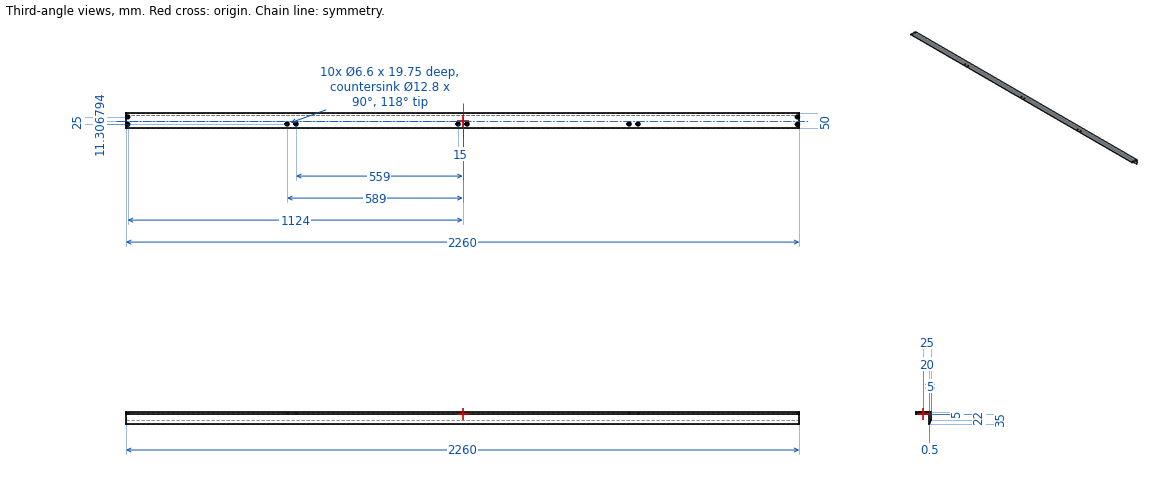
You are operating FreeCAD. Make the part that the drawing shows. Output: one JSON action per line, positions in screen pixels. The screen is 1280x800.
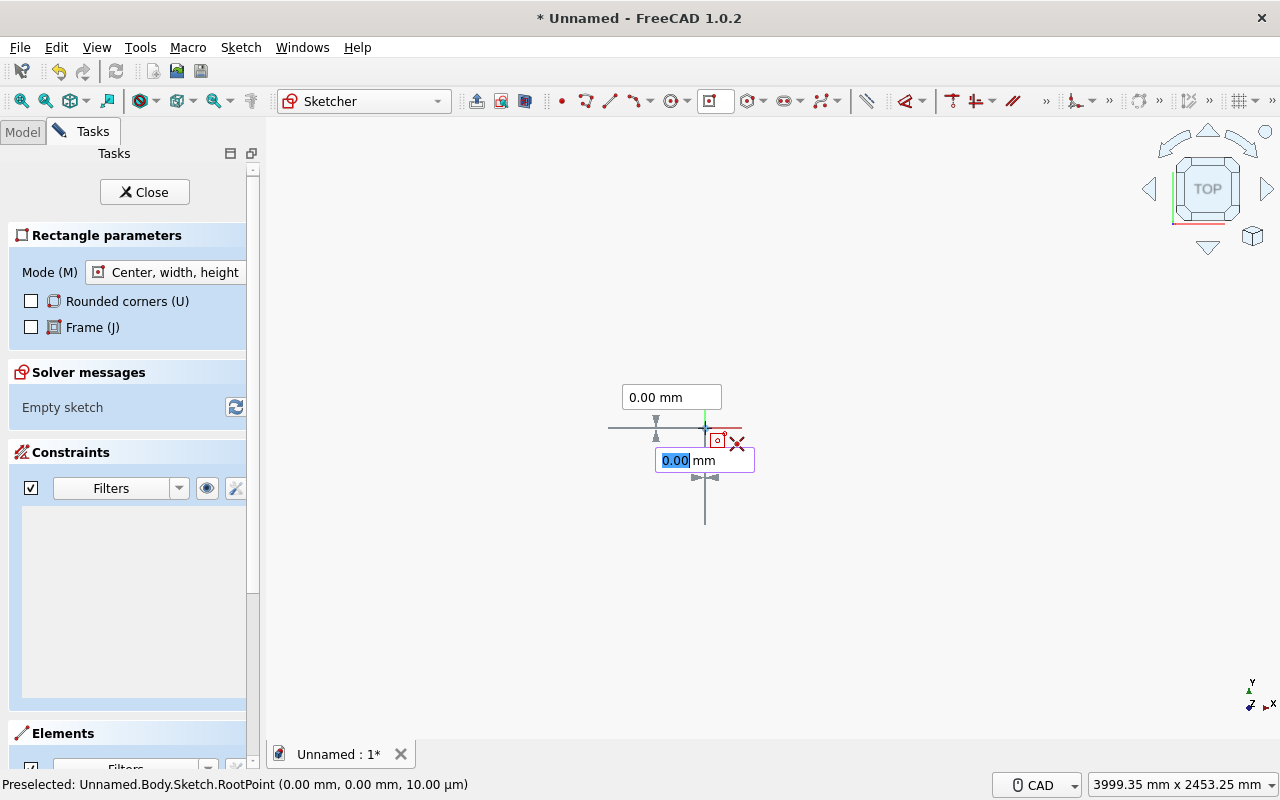
{"action": "scroll", "coordinate": [992, 422], "scroll_direction": "up", "scroll_amount": 5}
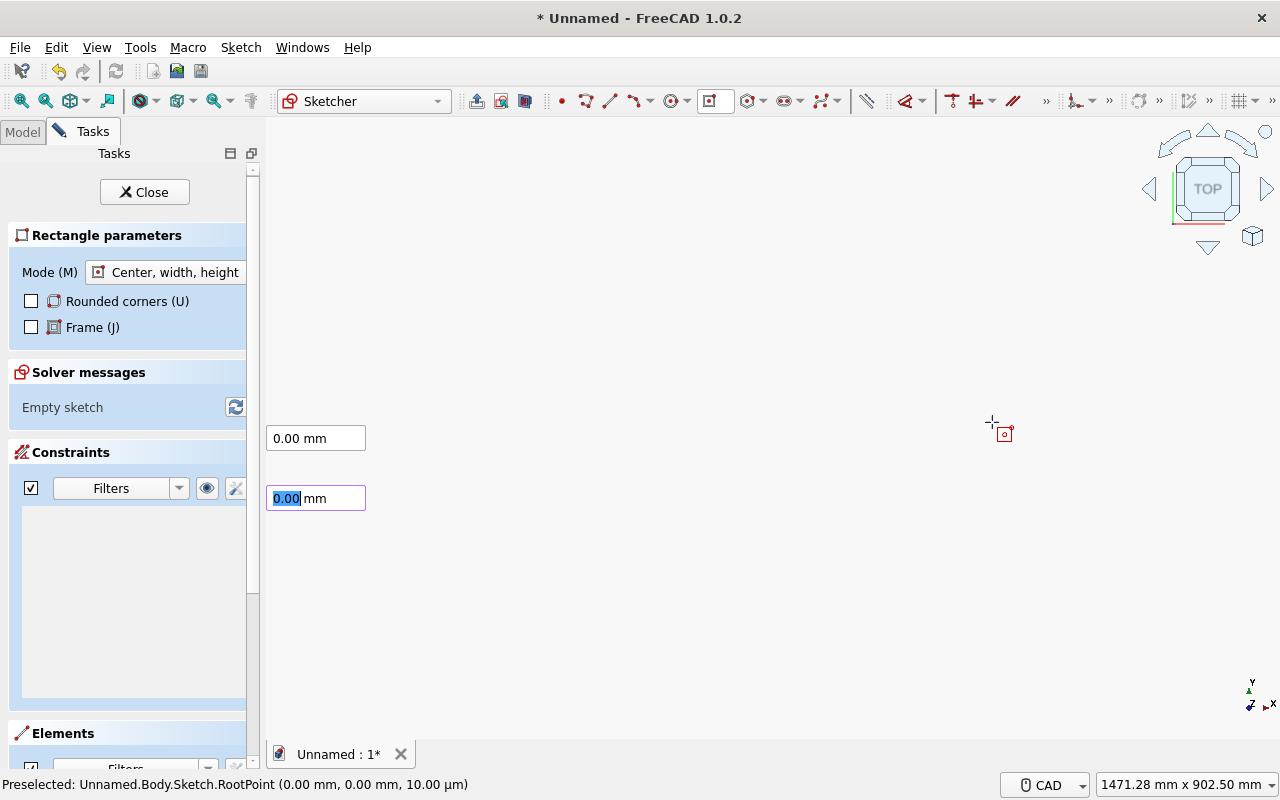
{"action": "left_click", "coordinate": [990, 422]}
{"action": "key", "text": "Escape"}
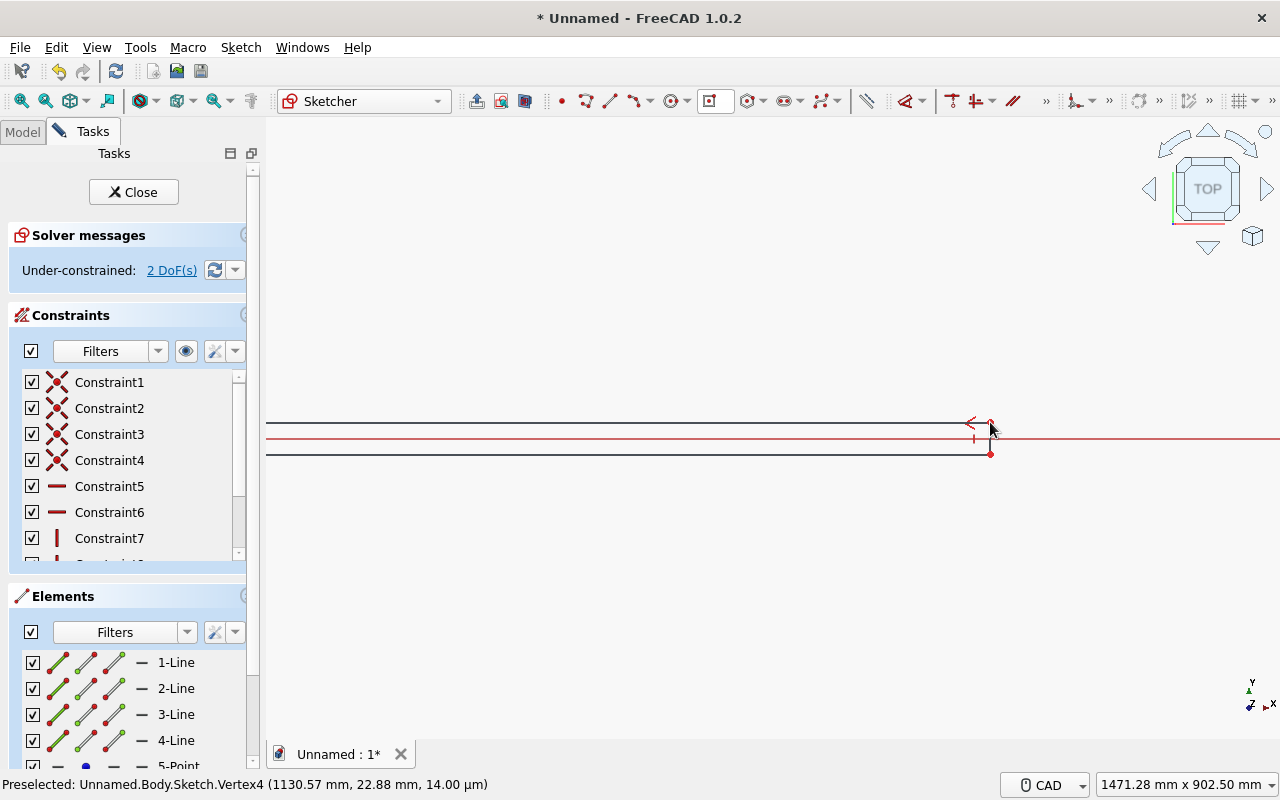
{"action": "left_click", "coordinate": [906, 102]}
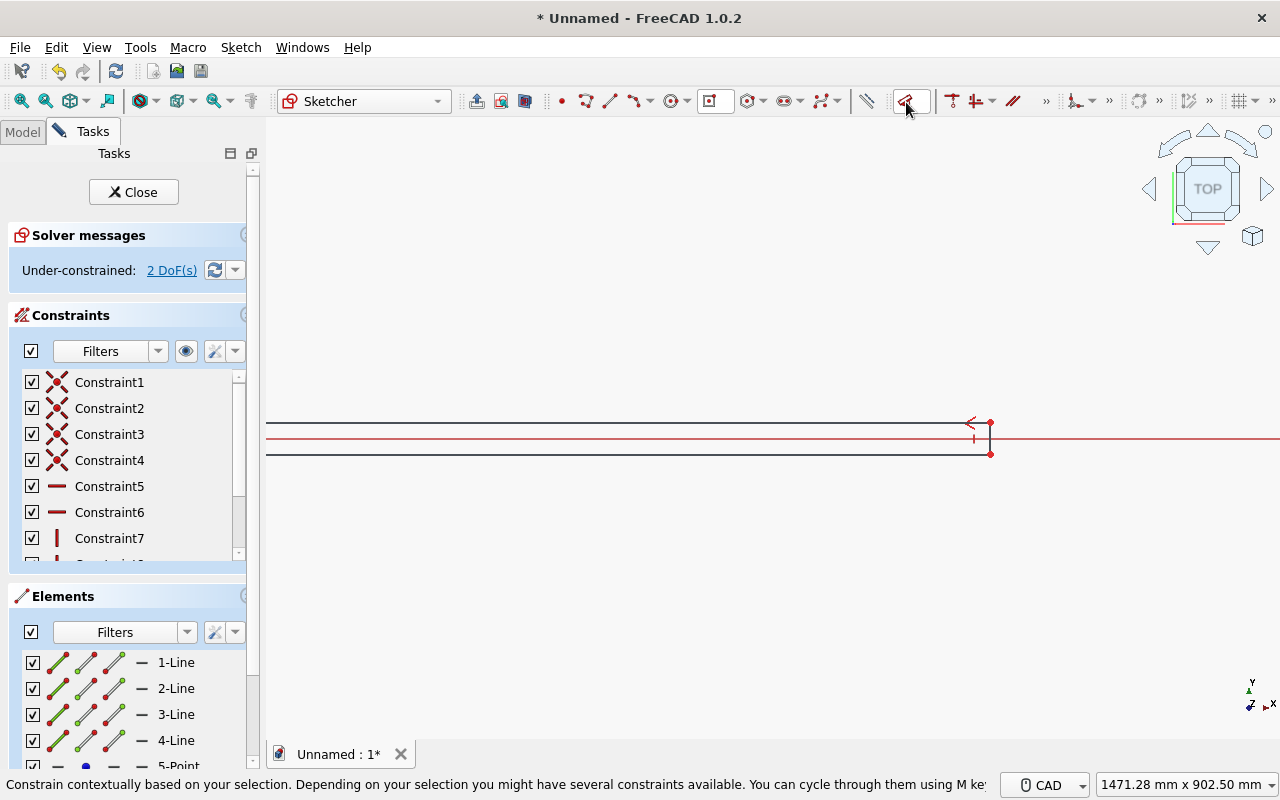
{"action": "left_click", "coordinate": [990, 442]}
{"action": "left_click", "coordinate": [1024, 432]}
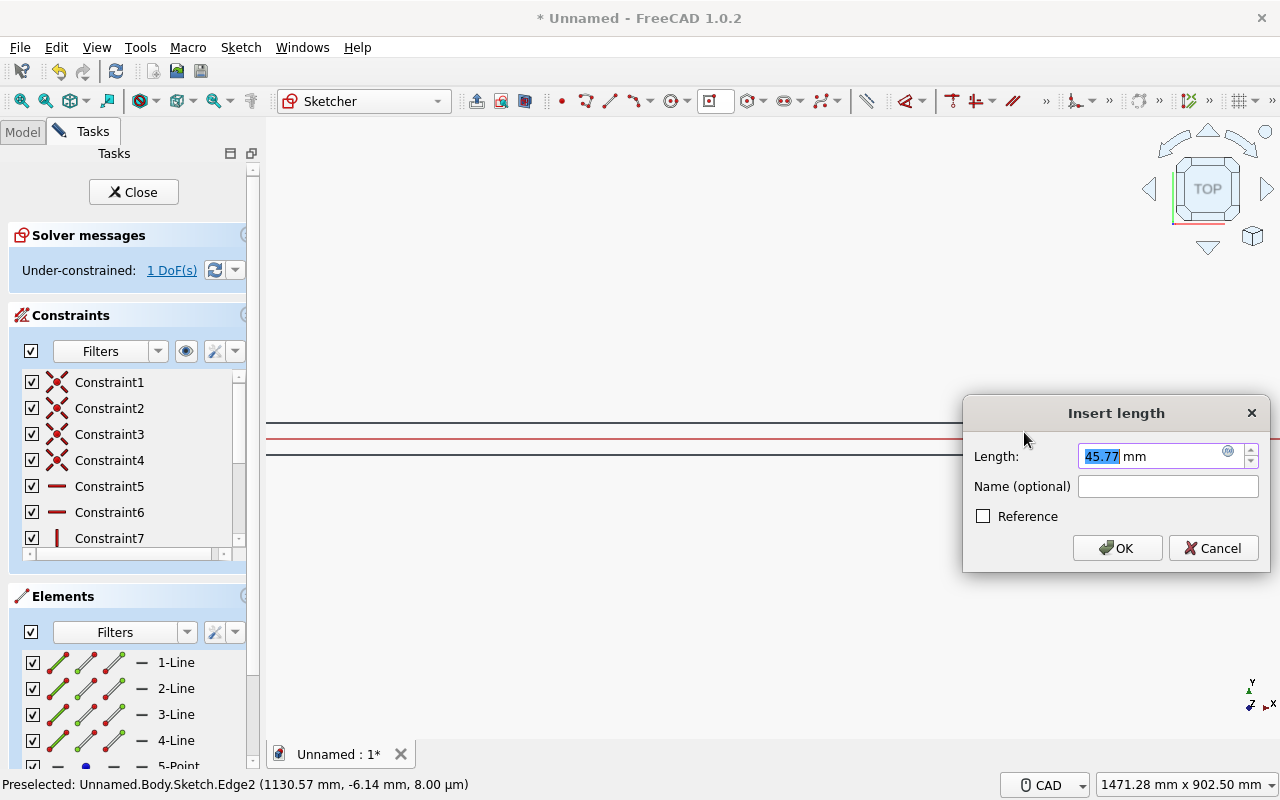
{"action": "type", "text": "50"}
{"action": "key", "text": "Return"}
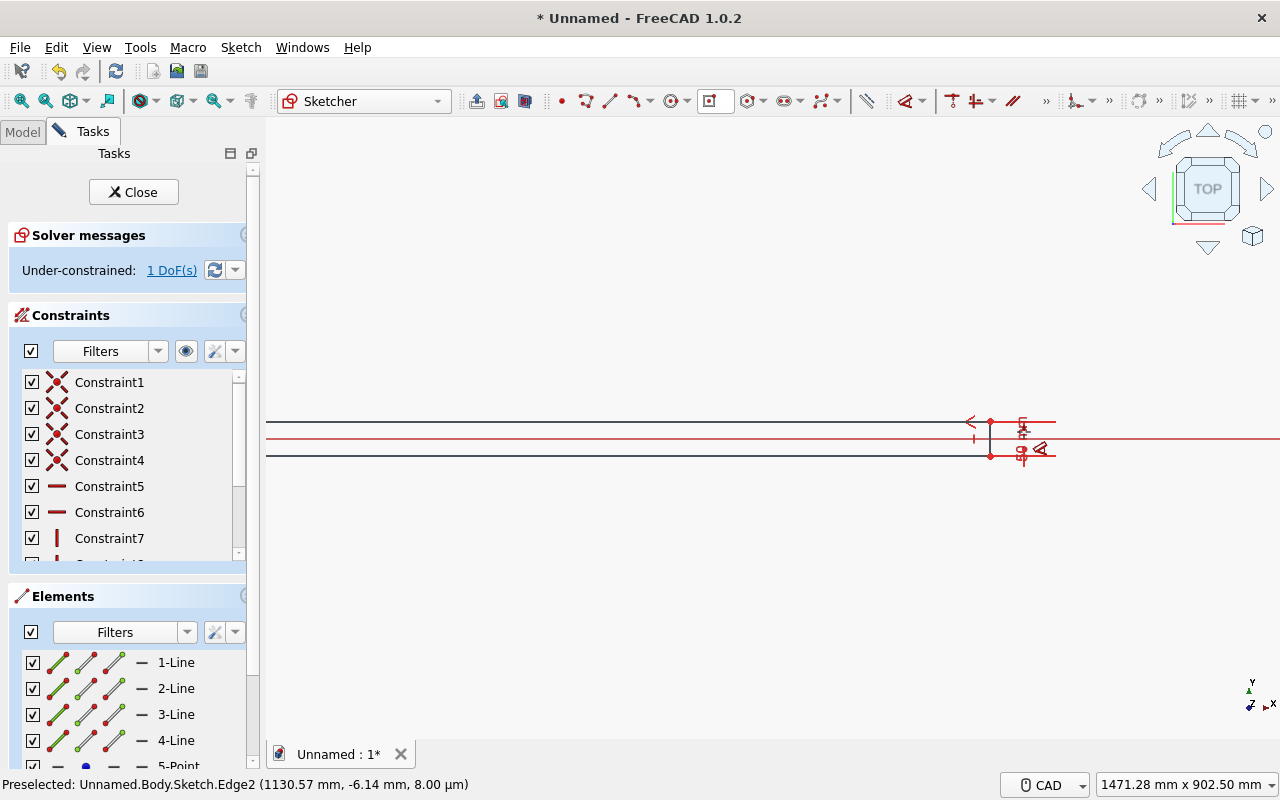
{"action": "left_click", "coordinate": [522, 456]}
{"action": "left_click", "coordinate": [642, 490]}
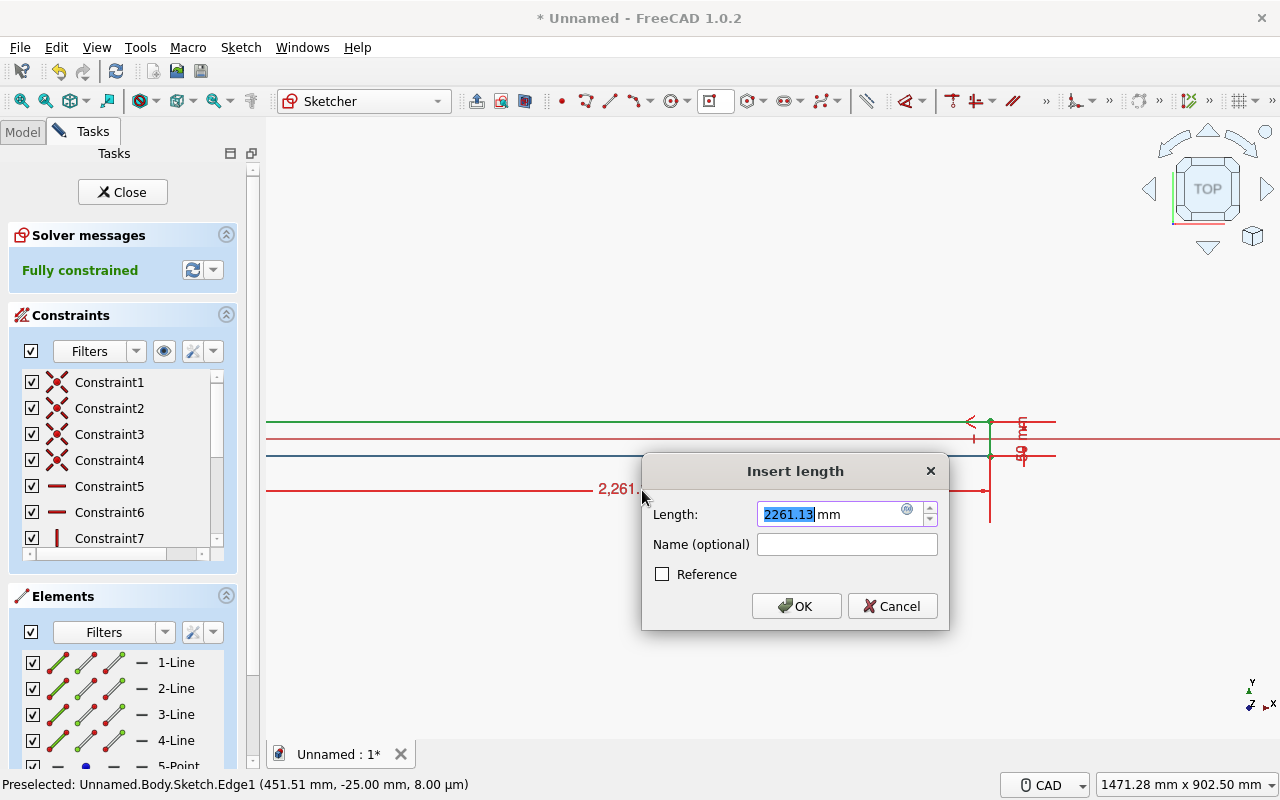
{"action": "type", "text": "2260"}
{"action": "key", "text": "Return"}
{"action": "key", "text": "Escape"}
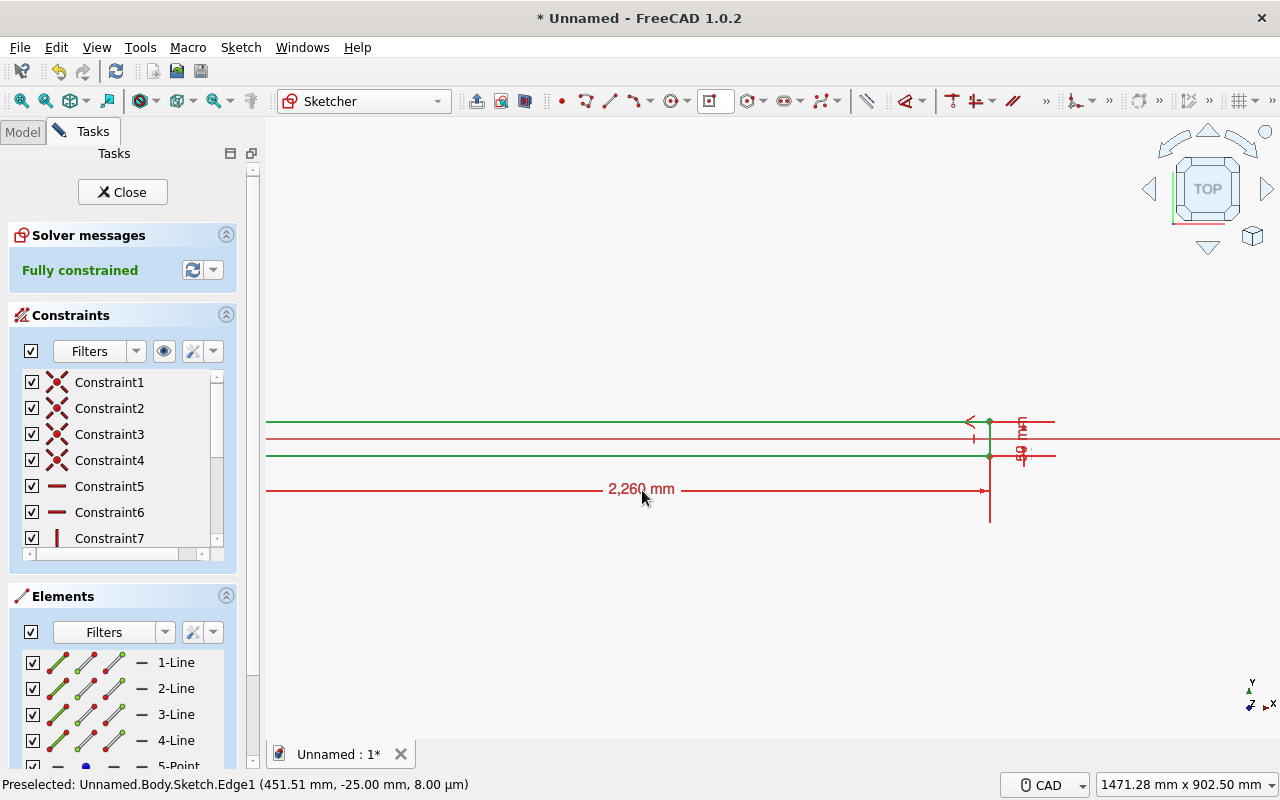
{"action": "left_click", "coordinate": [123, 192]}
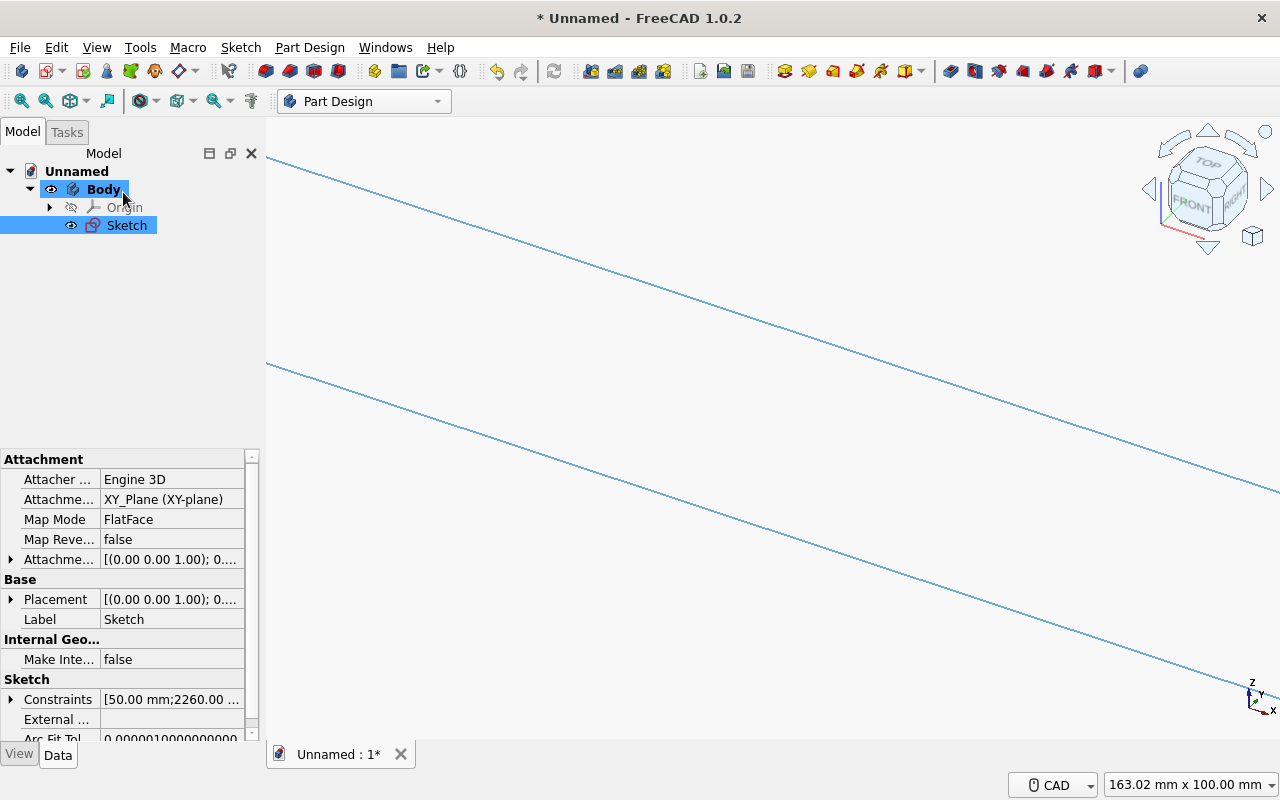
{"action": "left_click", "coordinate": [786, 72]}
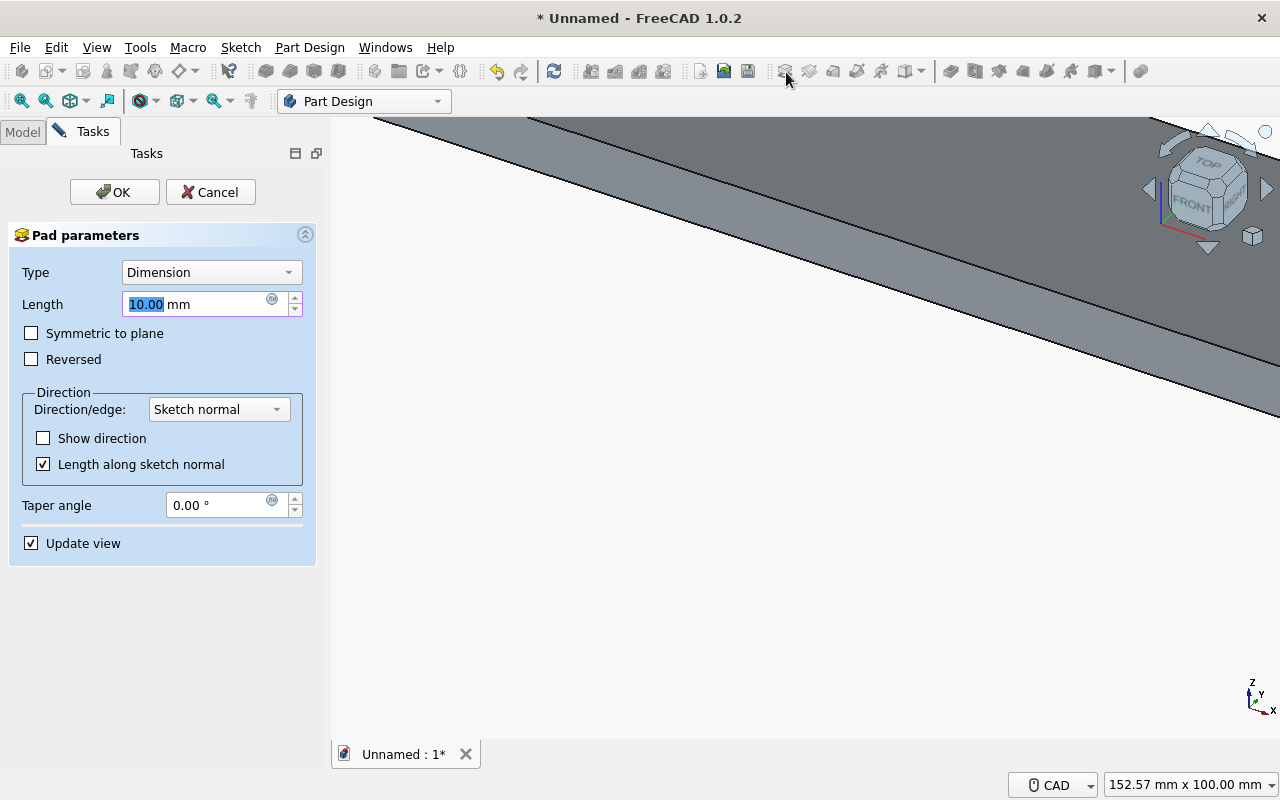
{"action": "type", "text": "5"}
{"action": "key", "text": "Tab"}